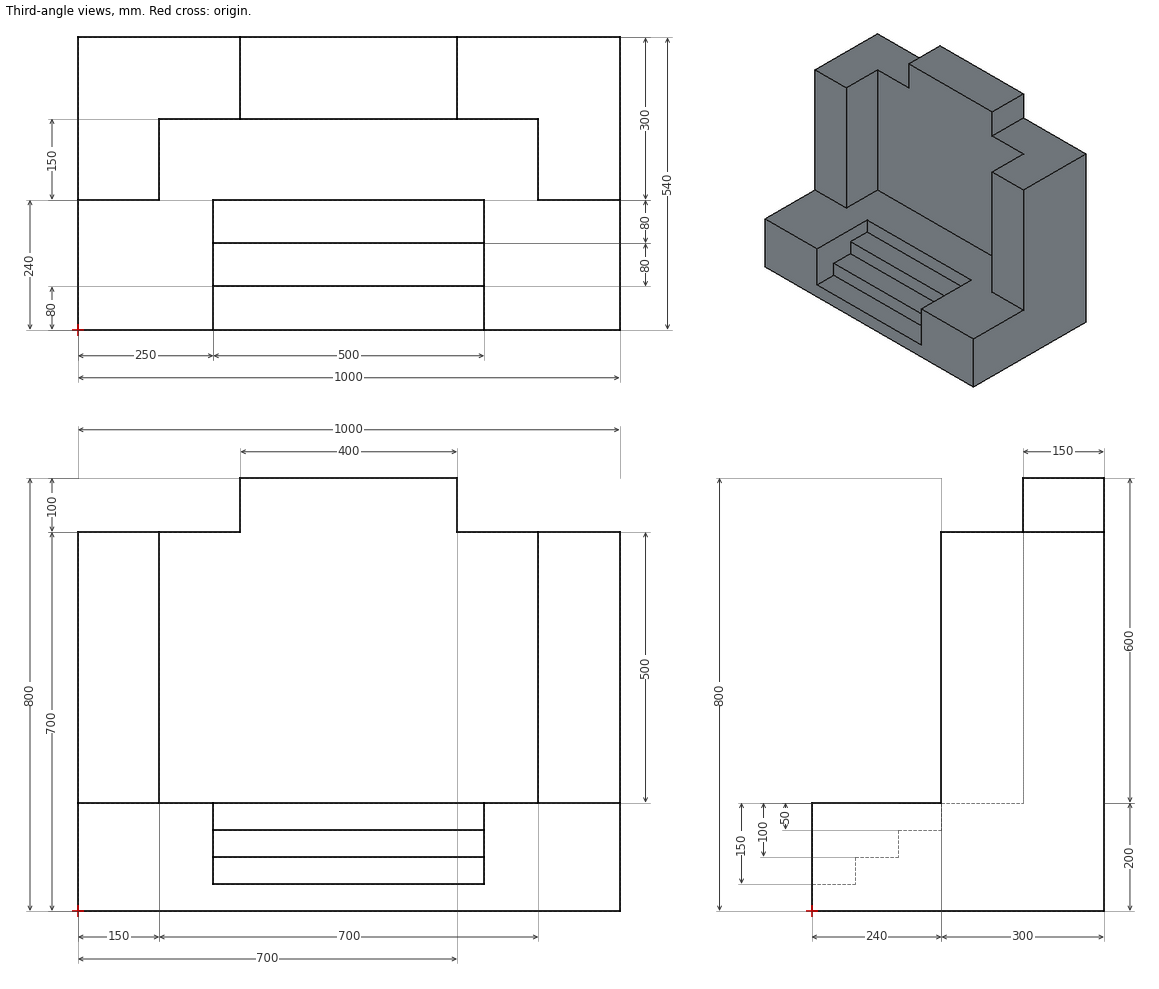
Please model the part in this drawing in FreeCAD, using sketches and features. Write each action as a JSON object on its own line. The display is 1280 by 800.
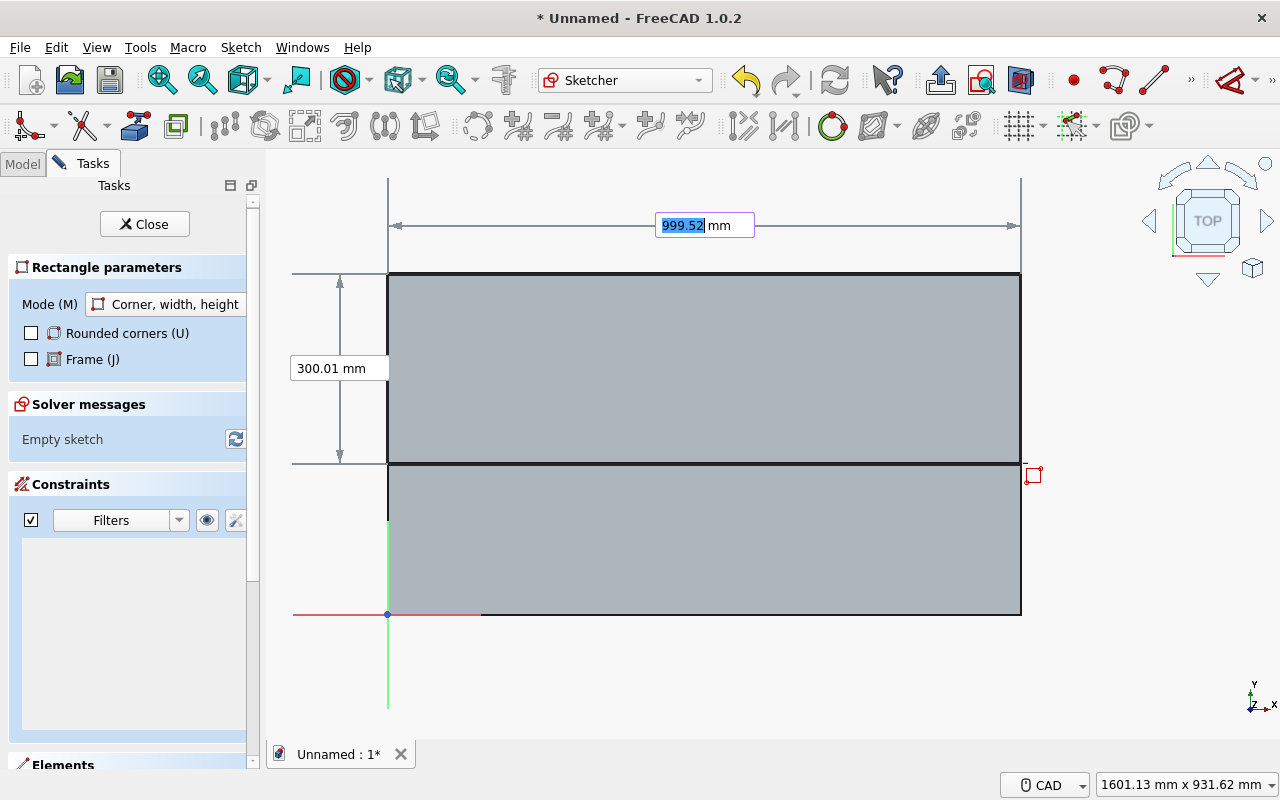
{"action": "type", "text": "1000"}
{"action": "key", "text": "Tab"}
{"action": "type", "text": "300"}
{"action": "key", "text": "Return"}
{"action": "key", "text": "Escape"}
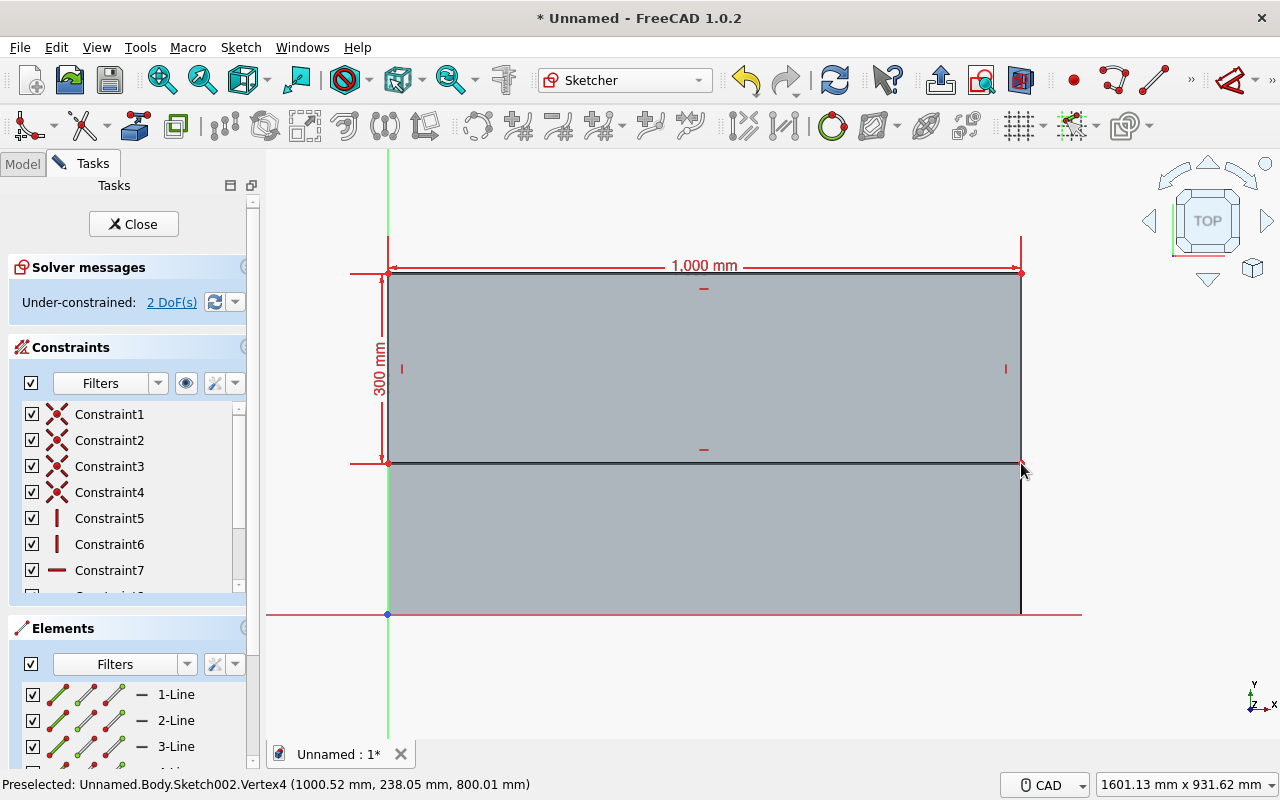
{"action": "left_click", "coordinate": [388, 274]}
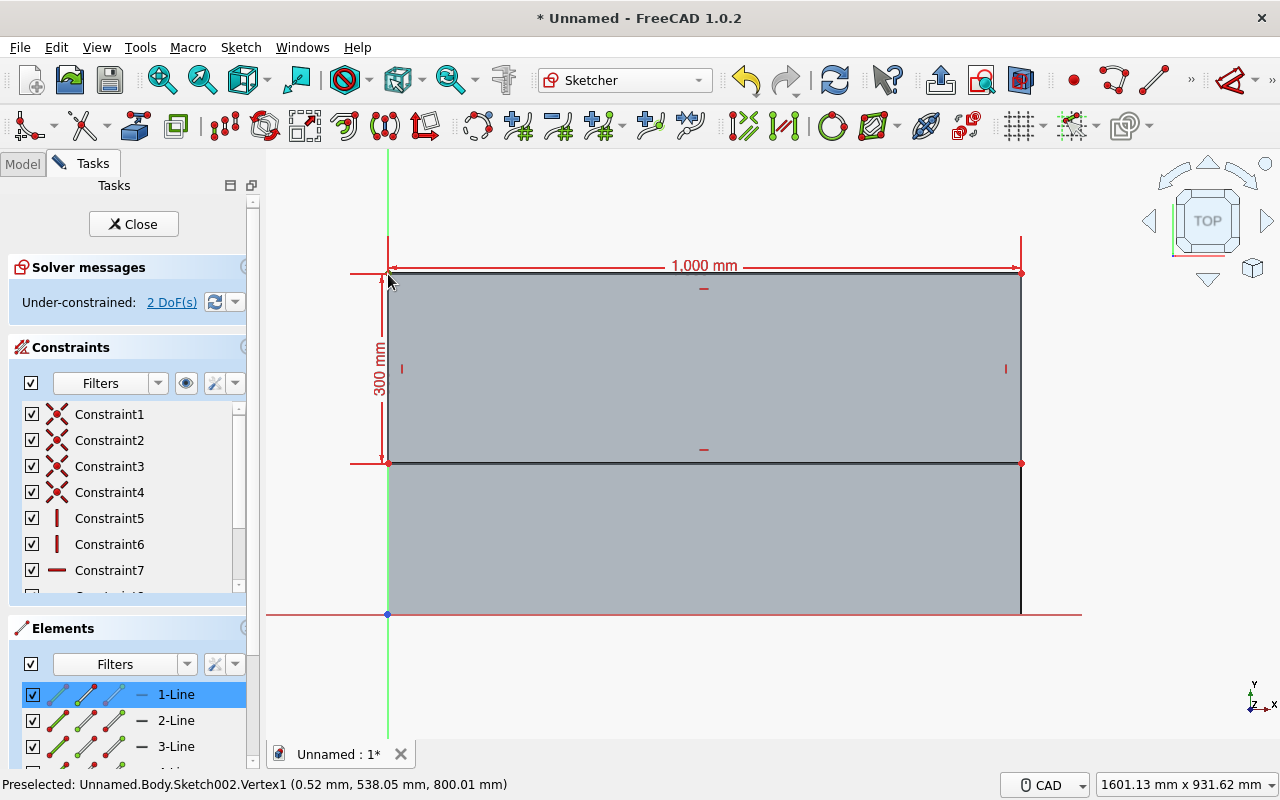
{"action": "left_click", "coordinate": [388, 673]}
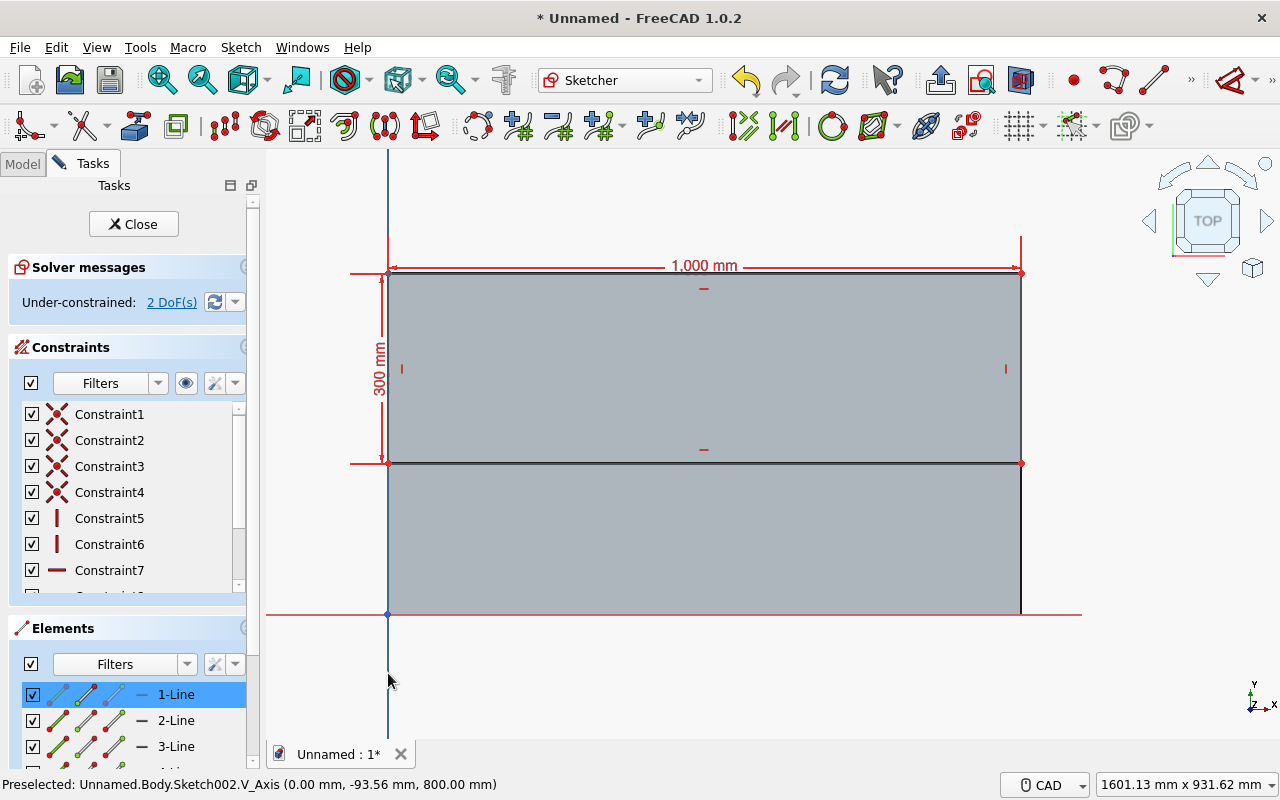
{"action": "key", "text": "c"}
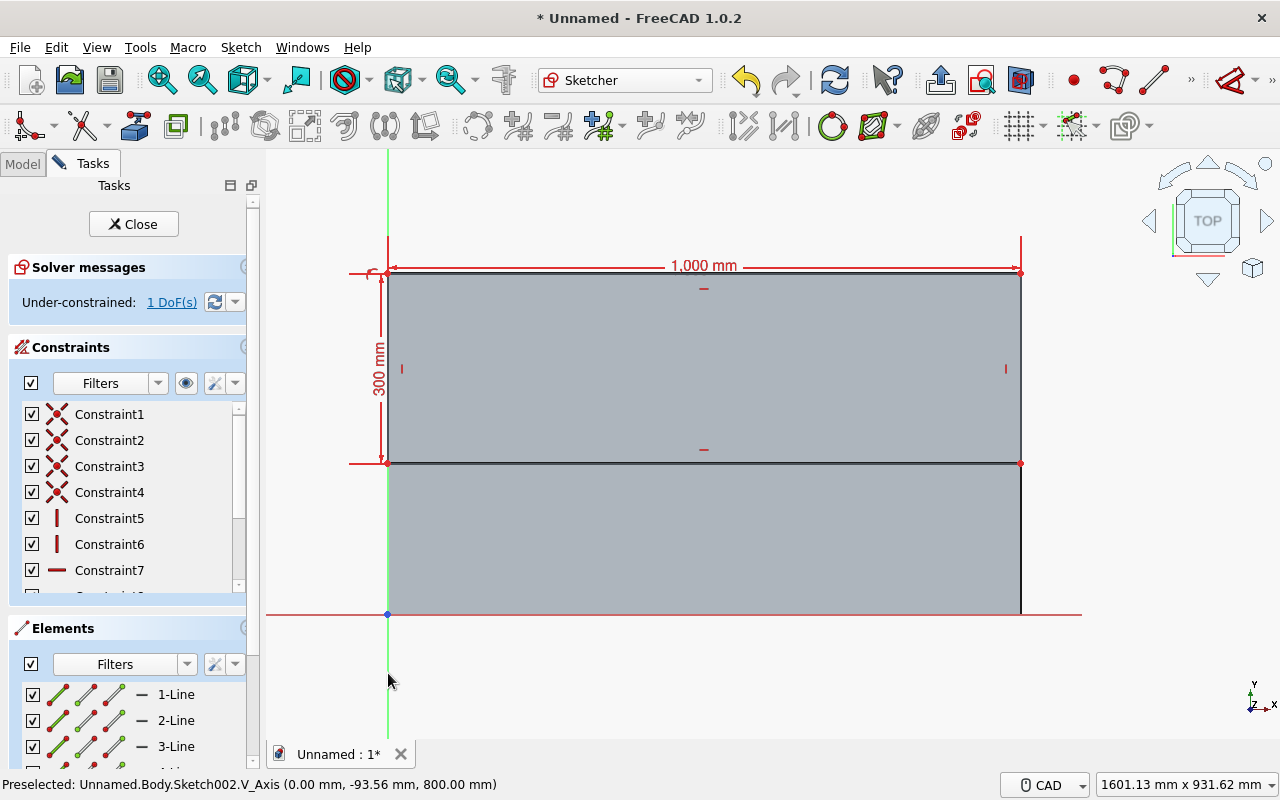
{"action": "left_click", "coordinate": [1230, 80]}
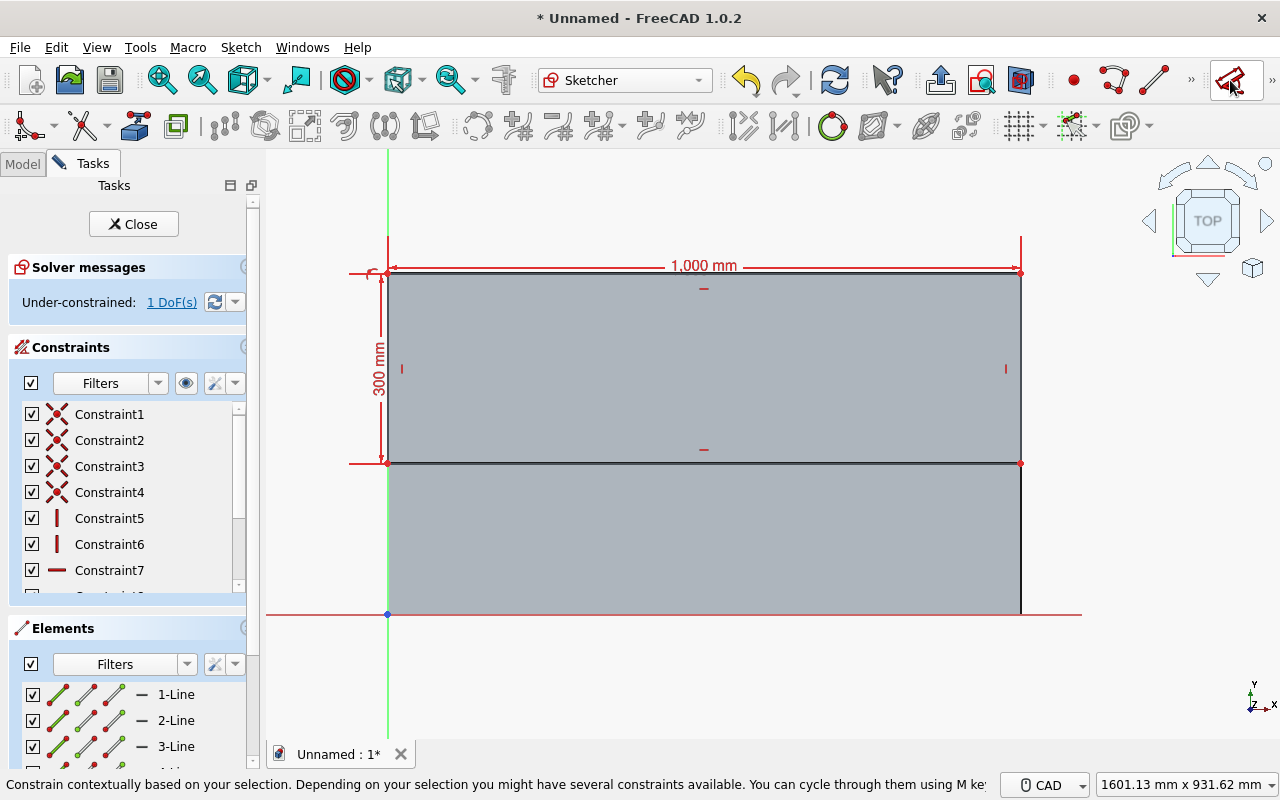
{"action": "left_click", "coordinate": [388, 274]}
{"action": "left_click", "coordinate": [354, 444]}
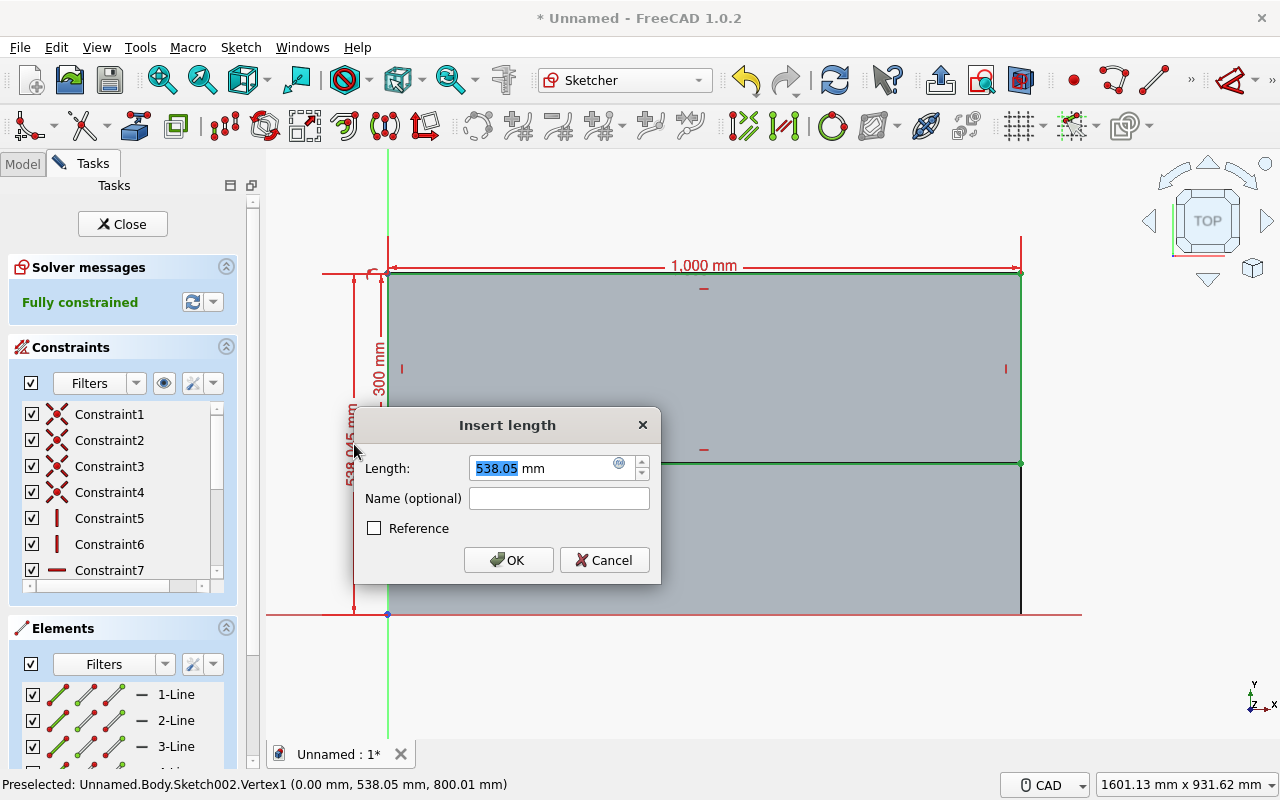
{"action": "type", "text": "540"}
{"action": "key", "text": "Return"}
{"action": "key", "text": "Escape"}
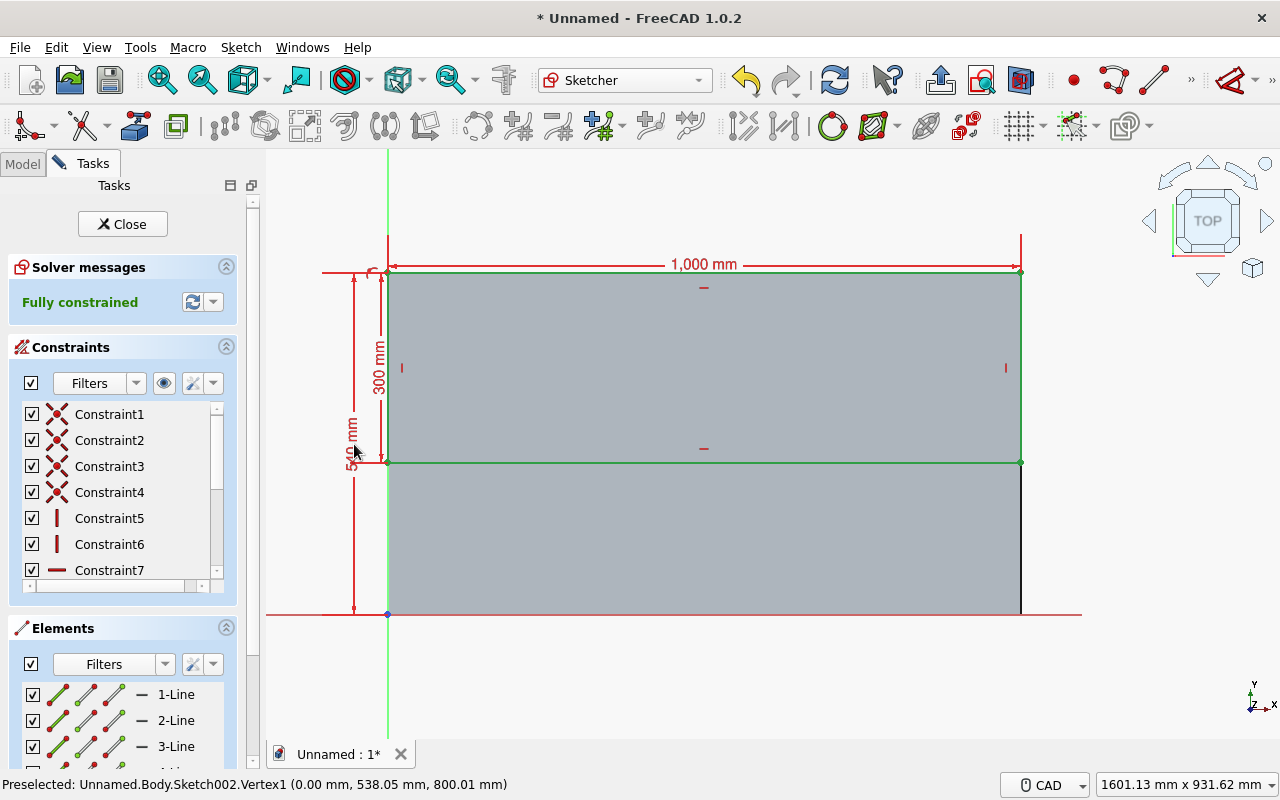
{"action": "left_click", "coordinate": [123, 224]}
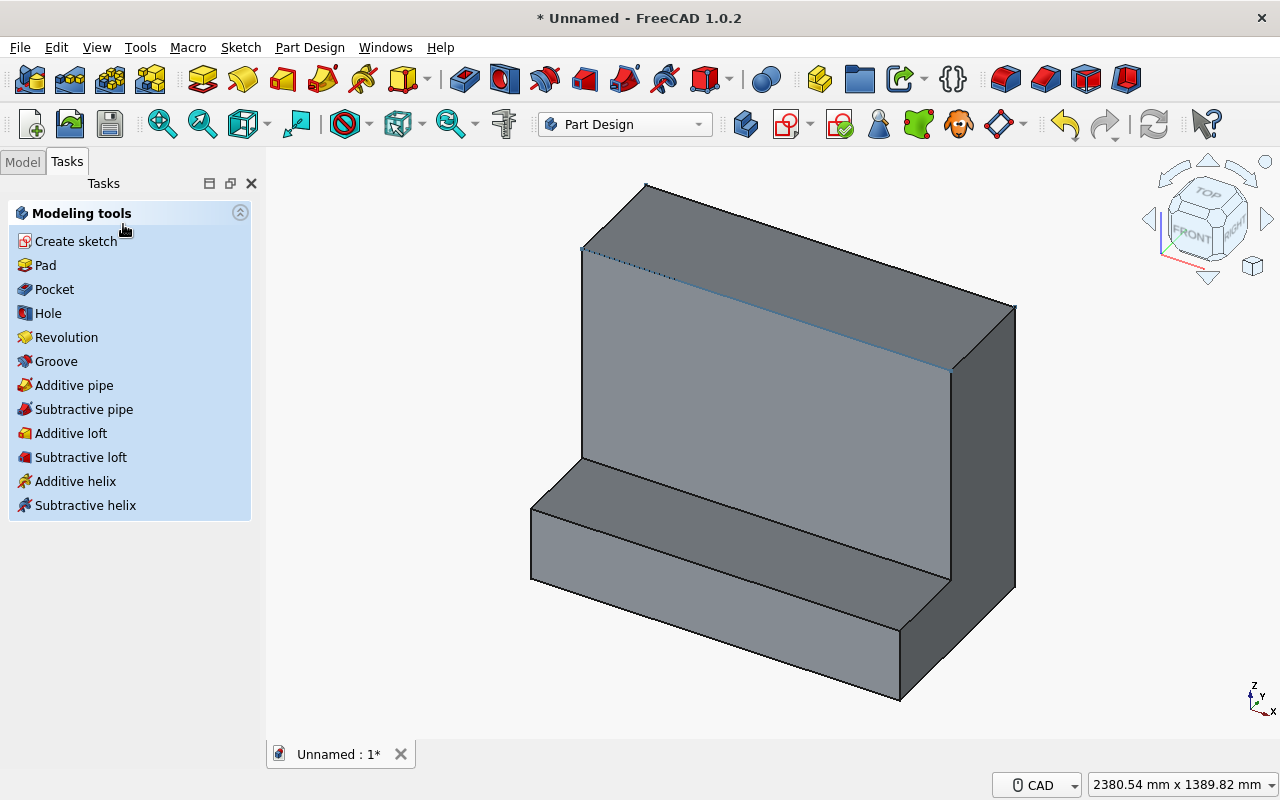
{"action": "left_click", "coordinate": [466, 80]}